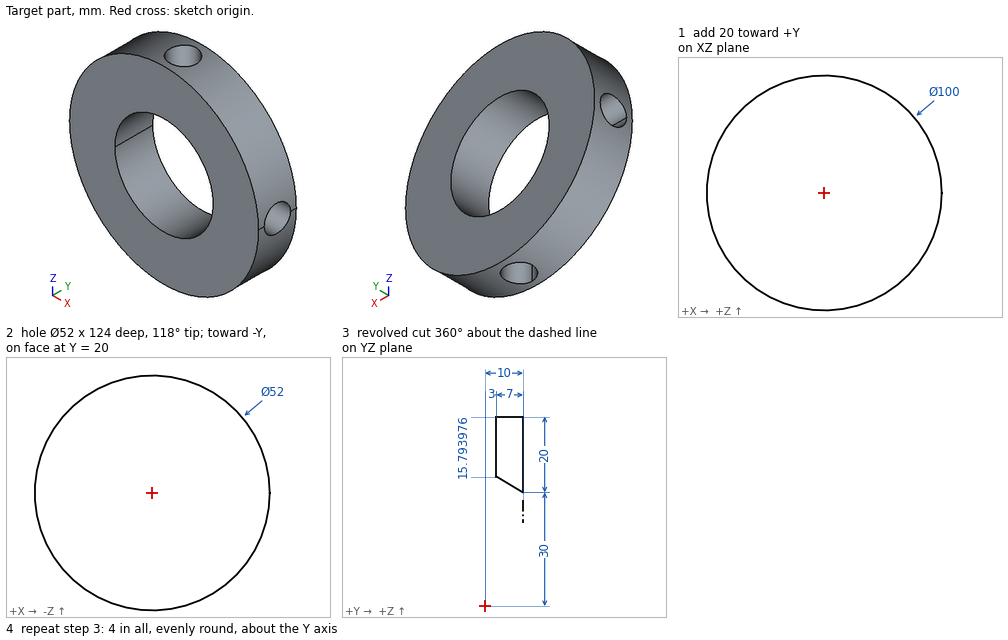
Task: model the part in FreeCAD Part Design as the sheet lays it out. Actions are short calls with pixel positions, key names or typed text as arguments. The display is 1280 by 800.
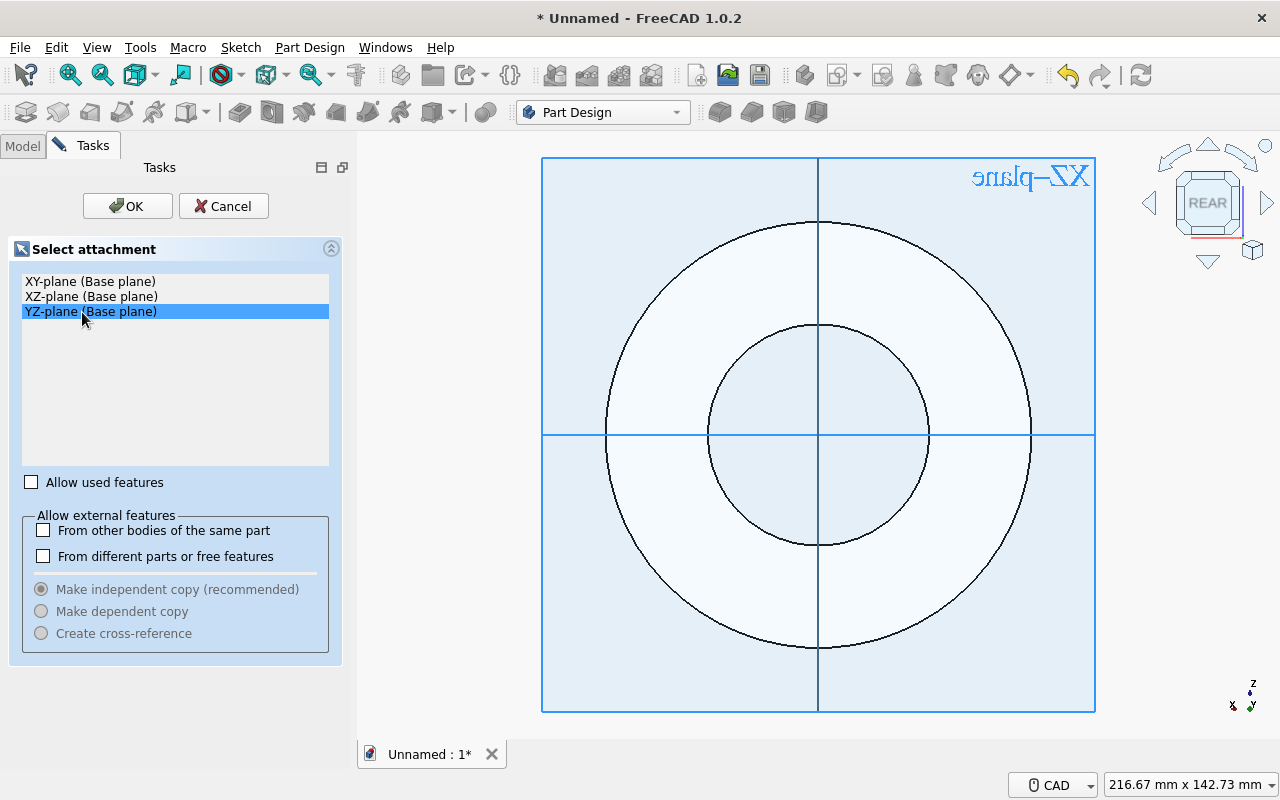
click(128, 206)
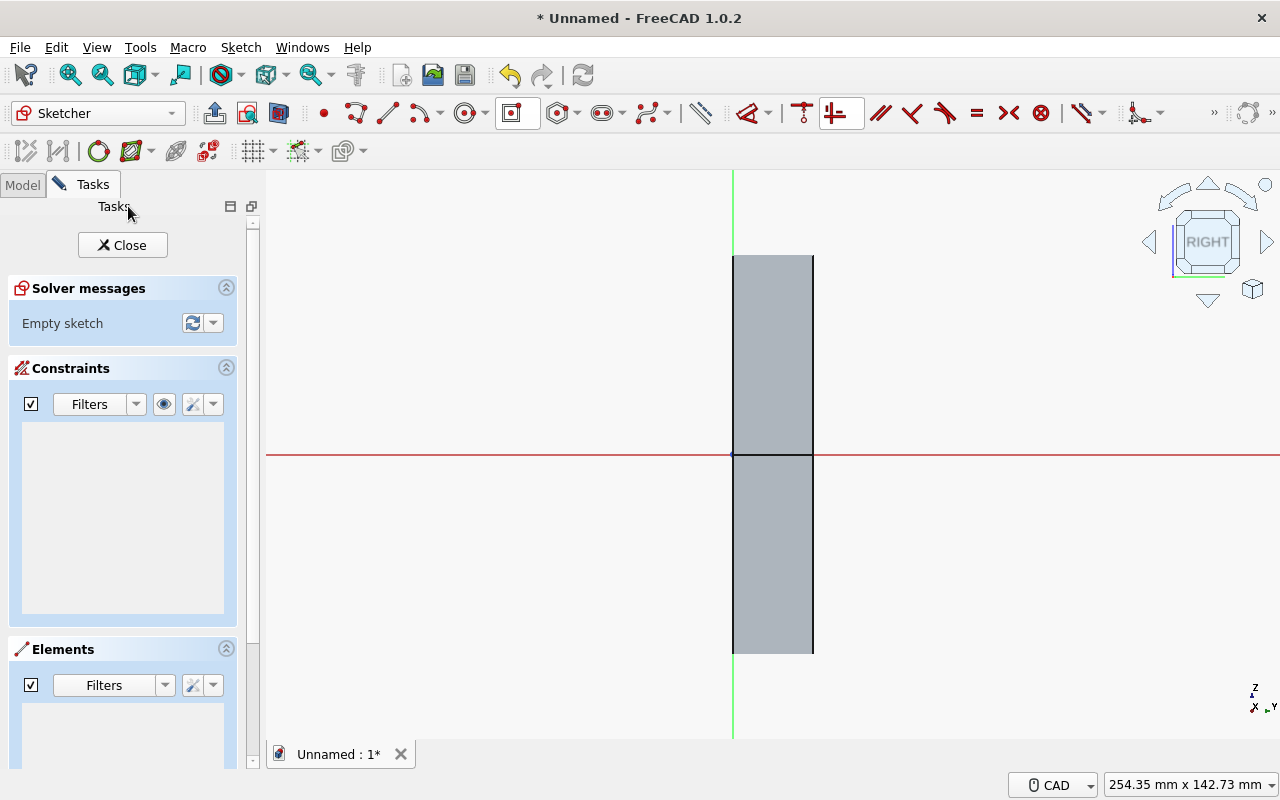
key(q)
key(s)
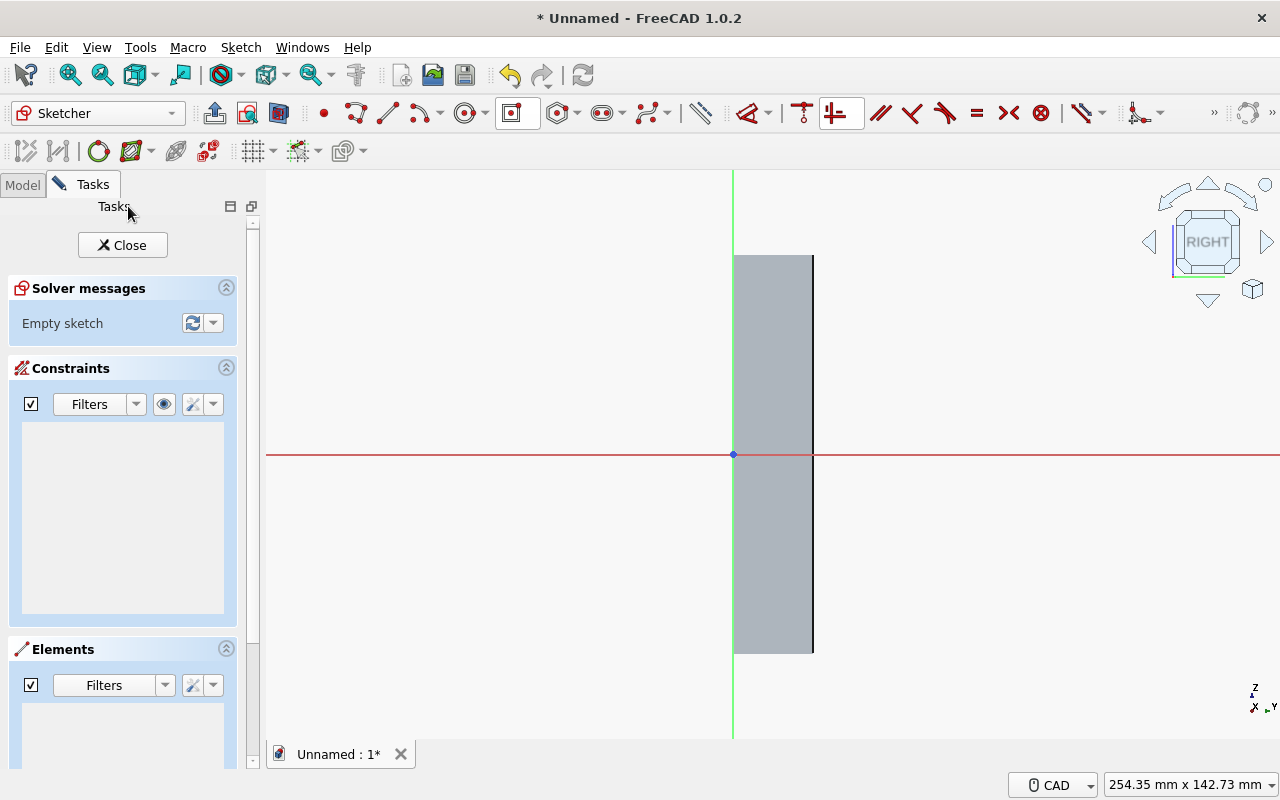
scroll(812, 234, up, 3)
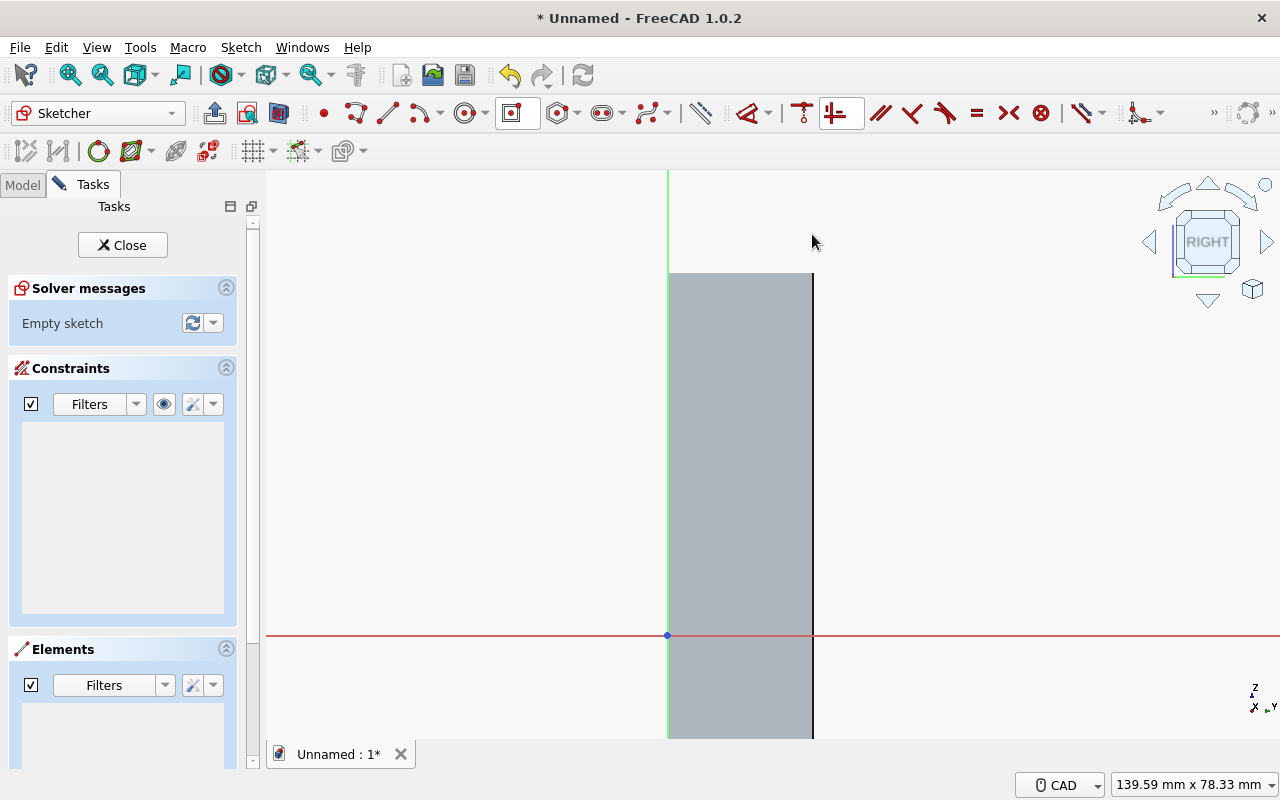
click(356, 114)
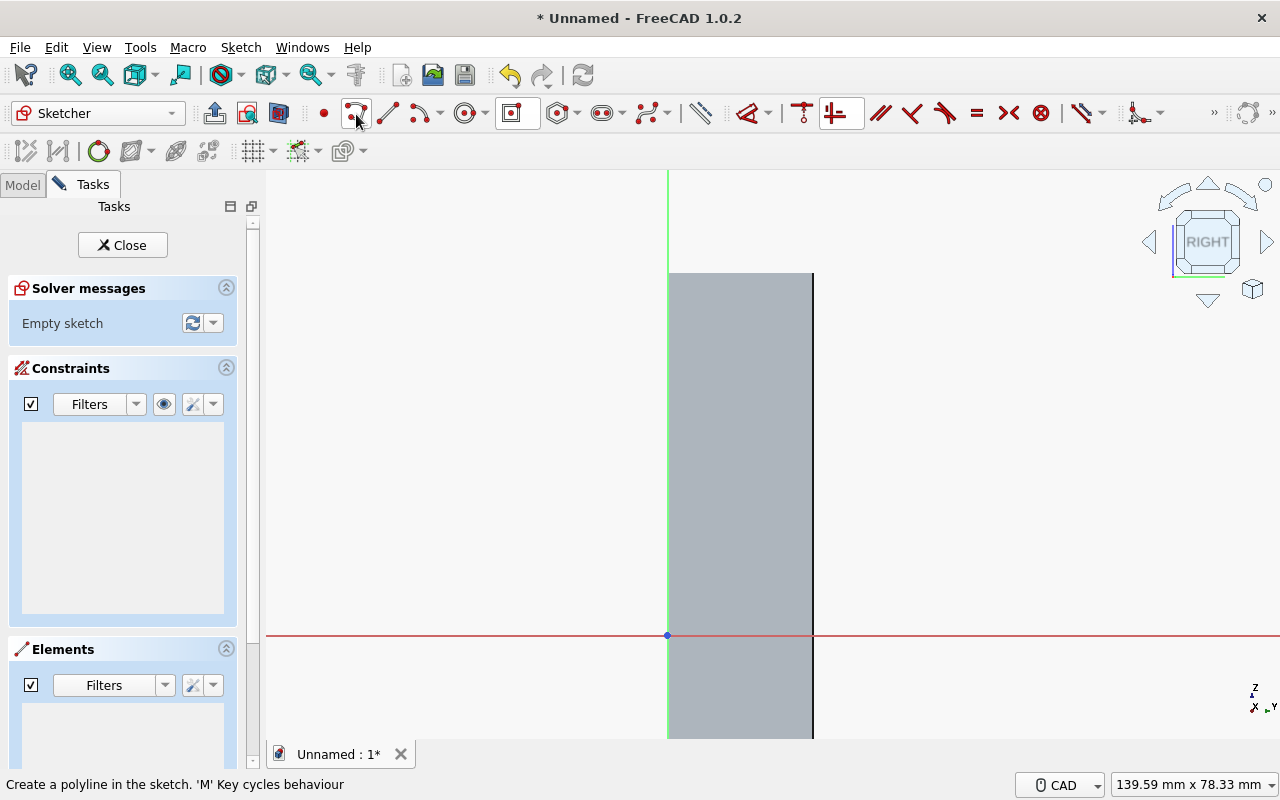
click(740, 418)
click(740, 272)
click(690, 272)
click(690, 387)
click(740, 419)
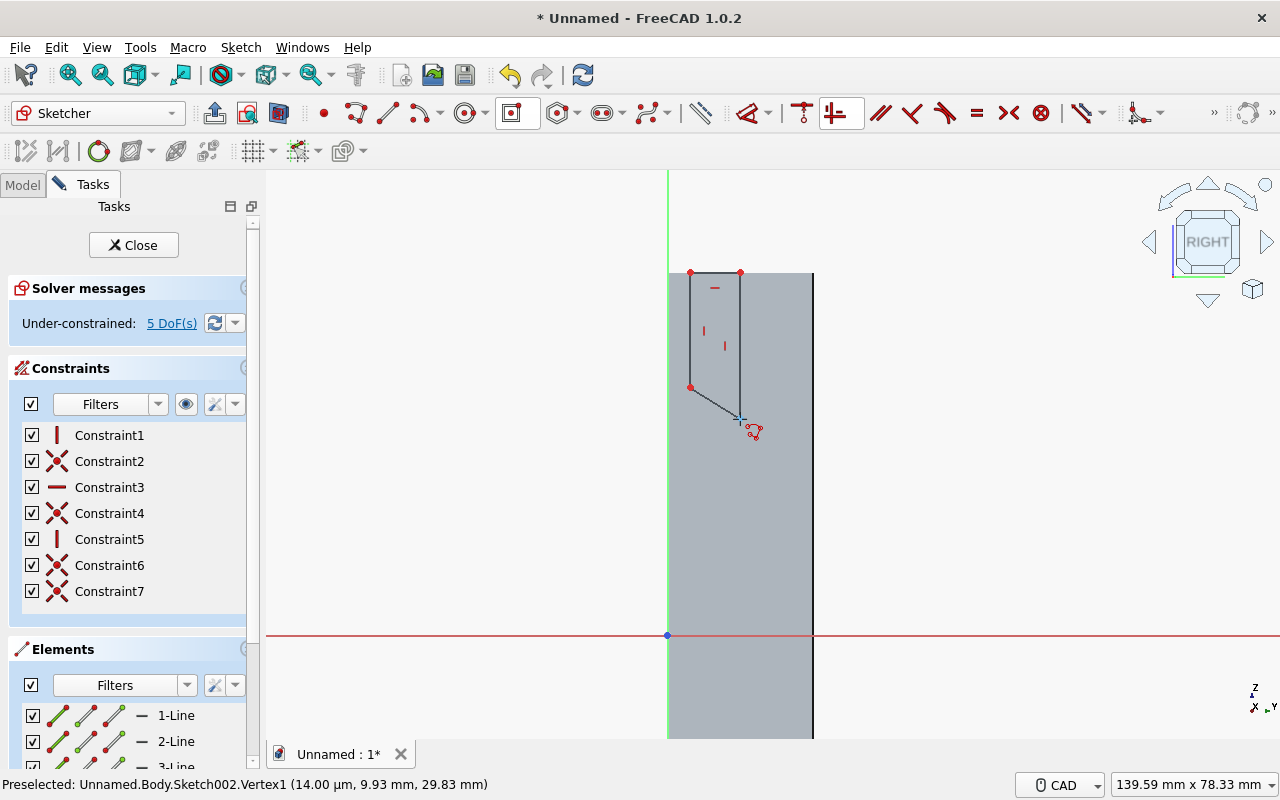
key(g)
key(l)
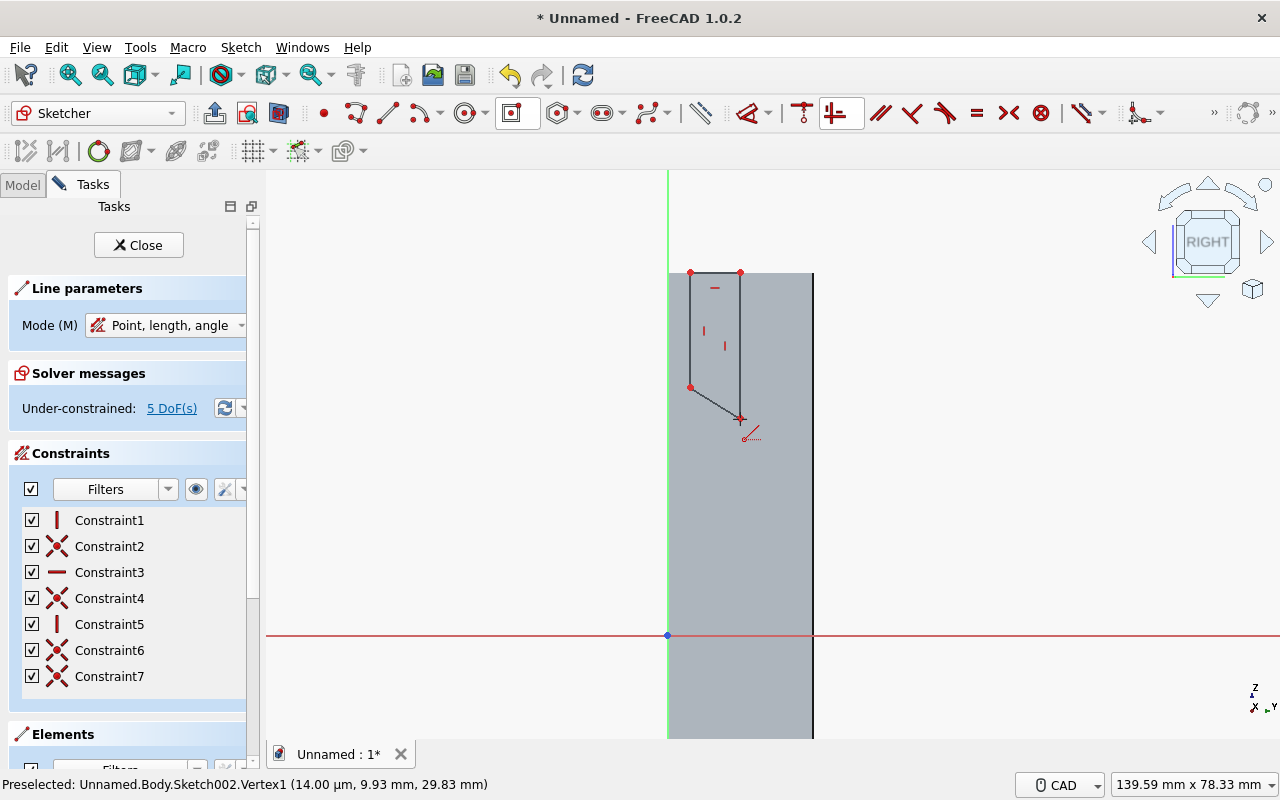
click(740, 432)
click(740, 476)
key(Escape)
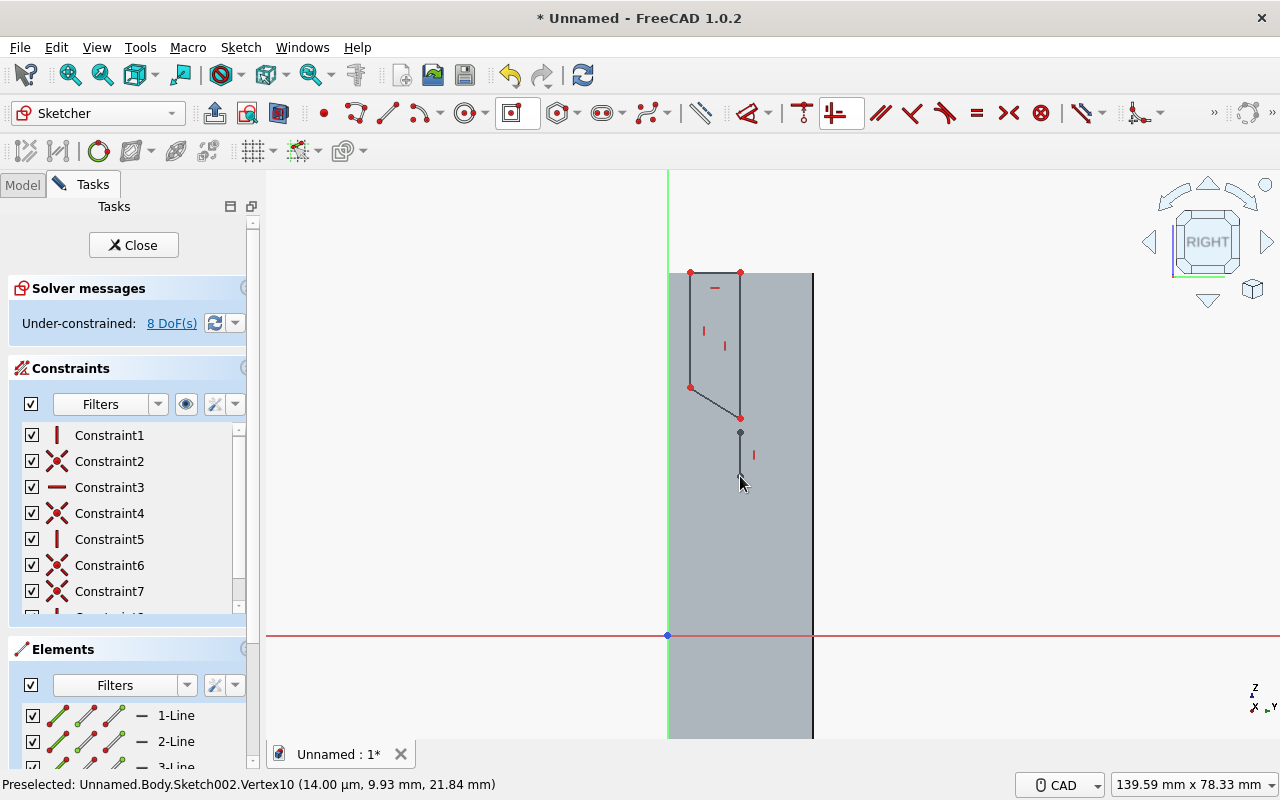
click(740, 446)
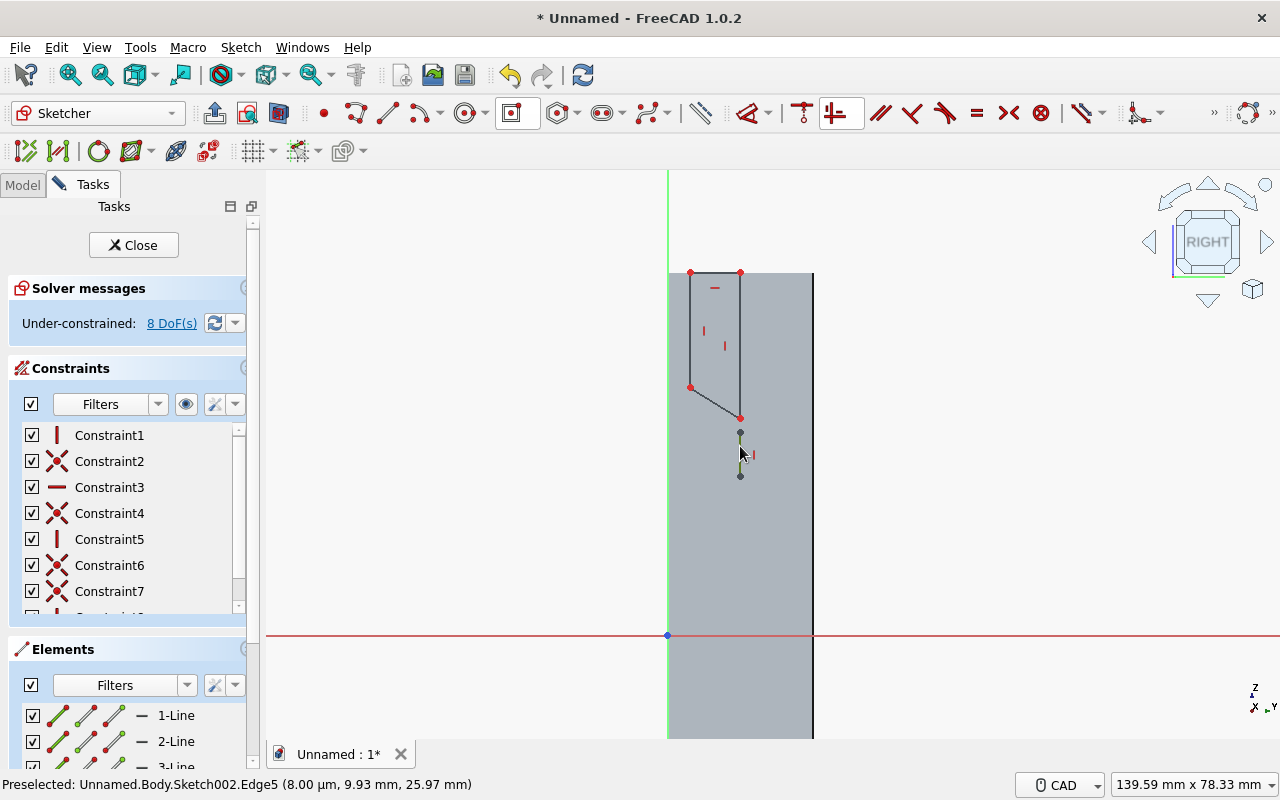
click(702, 114)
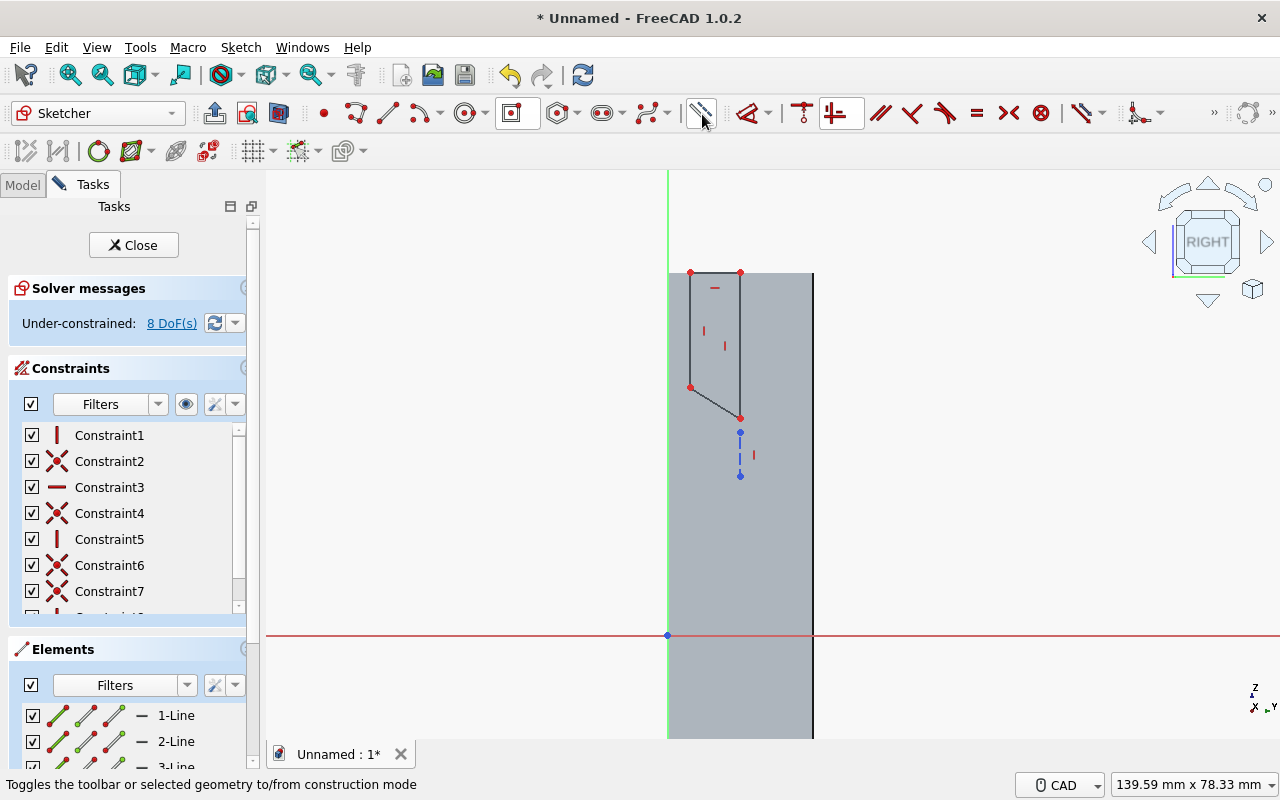
key(d)